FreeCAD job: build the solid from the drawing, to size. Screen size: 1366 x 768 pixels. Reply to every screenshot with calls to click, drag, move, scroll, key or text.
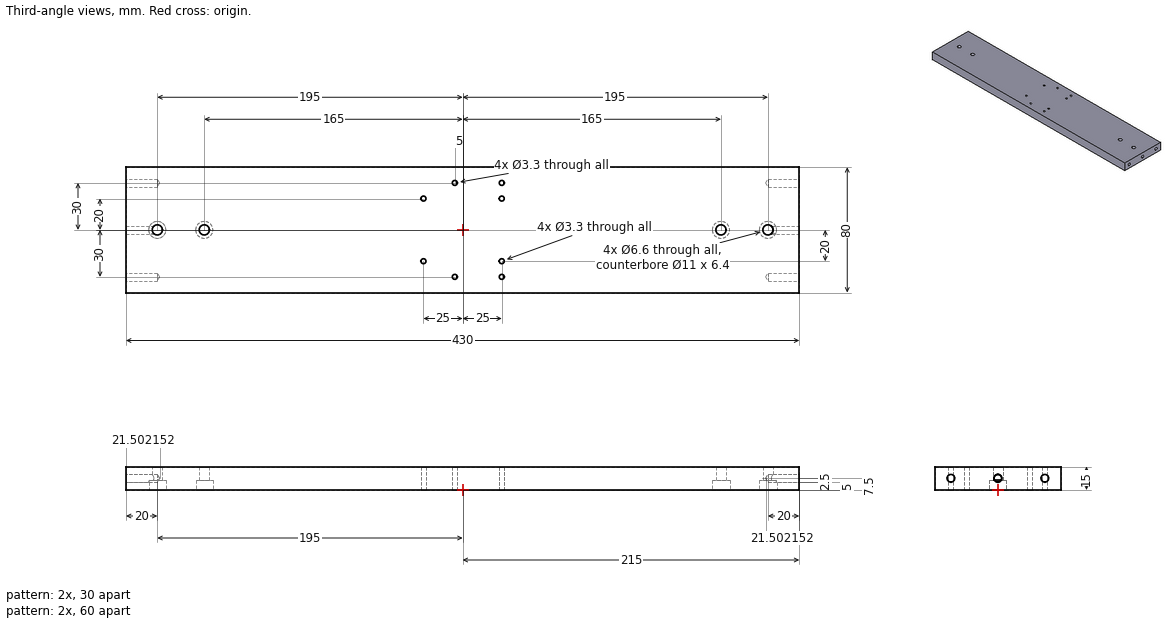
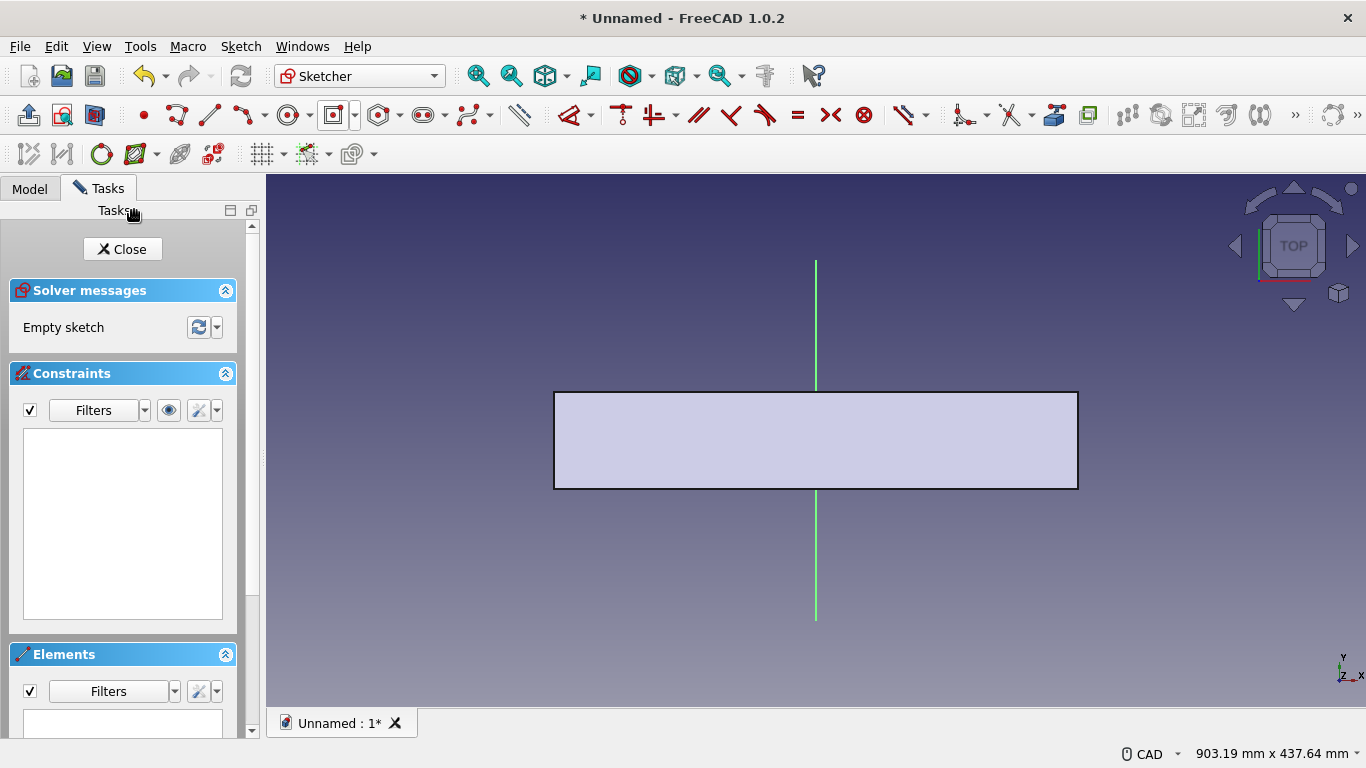
click(95, 116)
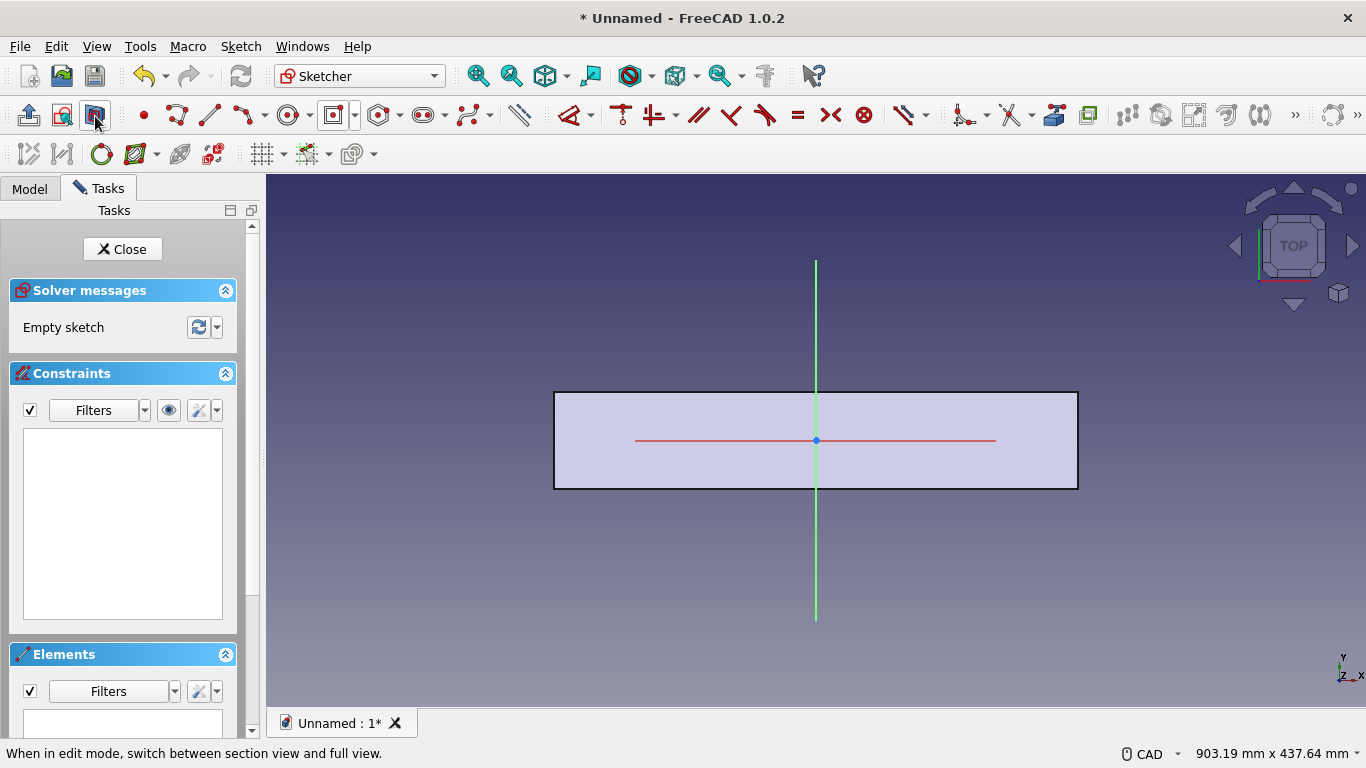
scroll(830, 440, up, 9)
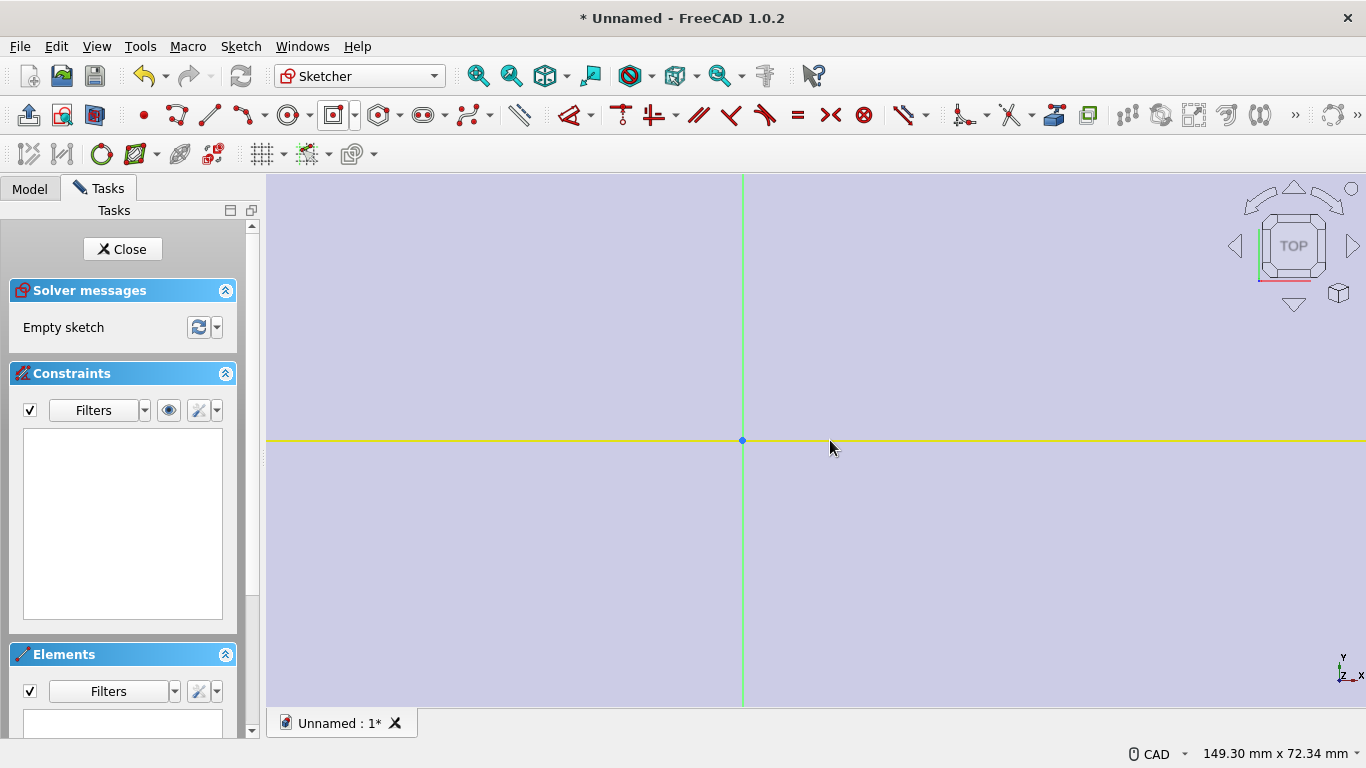
key(g)
key(c)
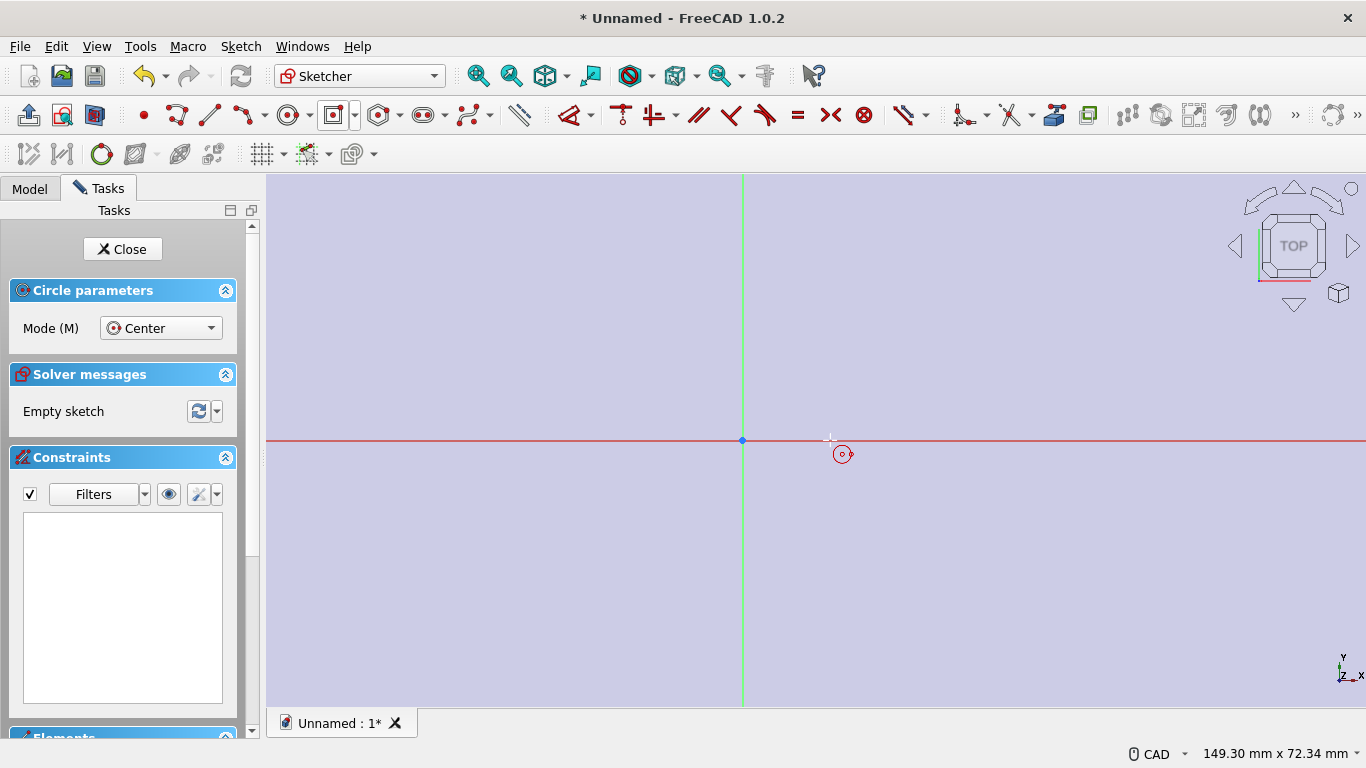
scroll(927, 588, up, 4)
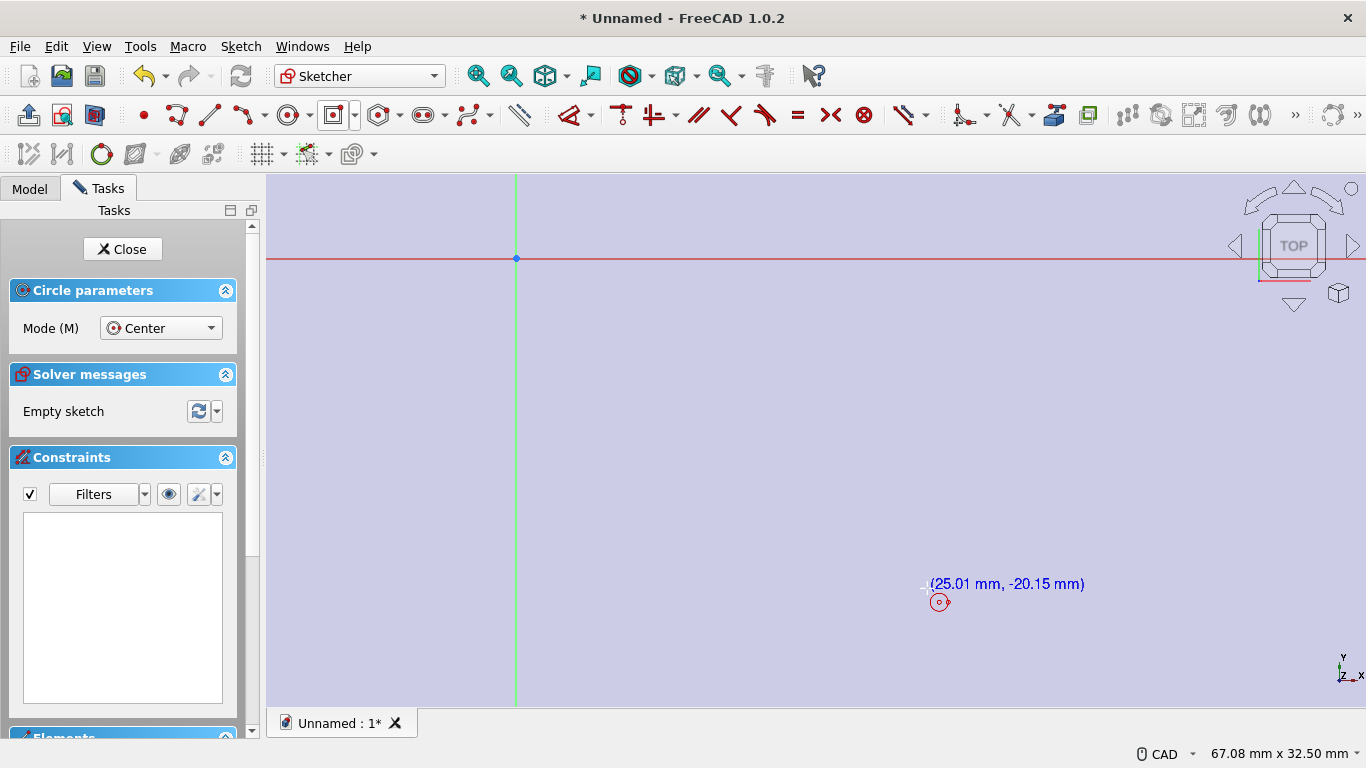
click(926, 587)
click(945, 568)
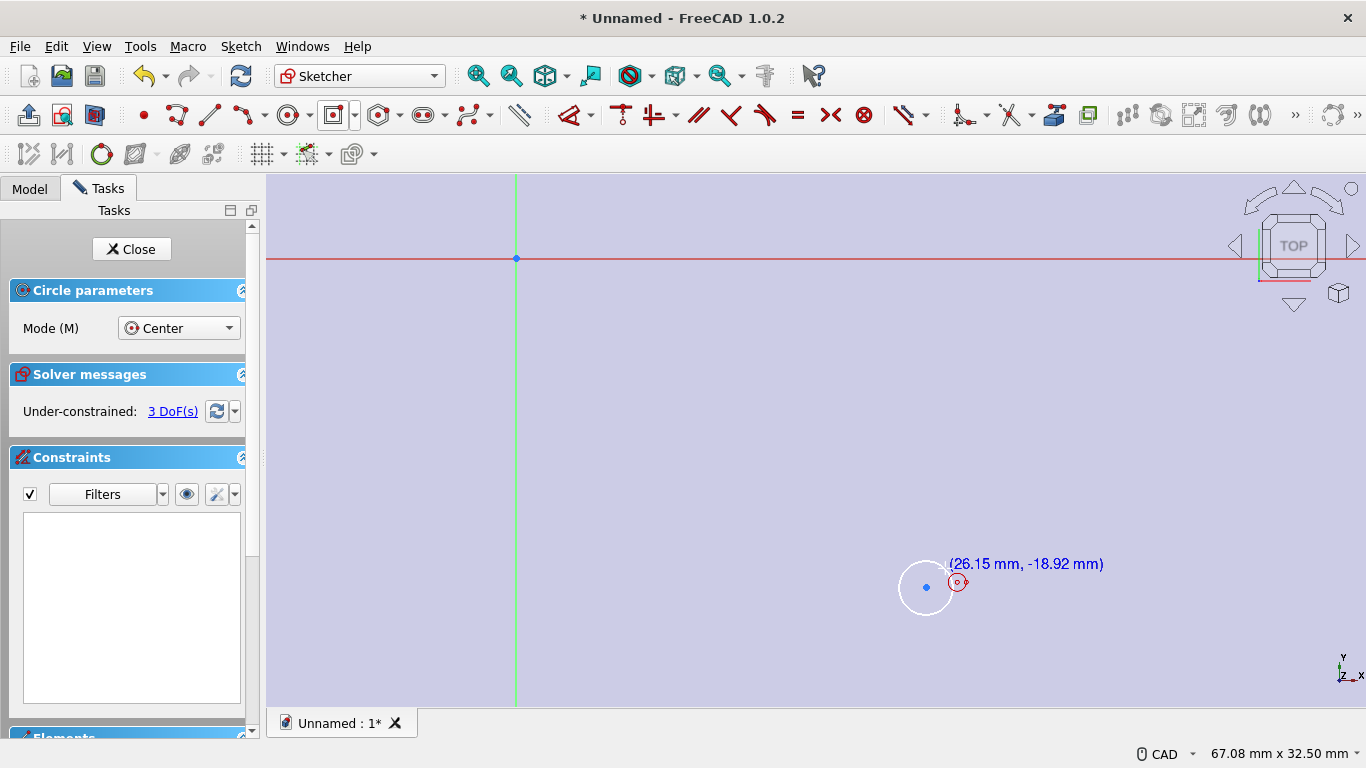
scroll(936, 589, down, 4)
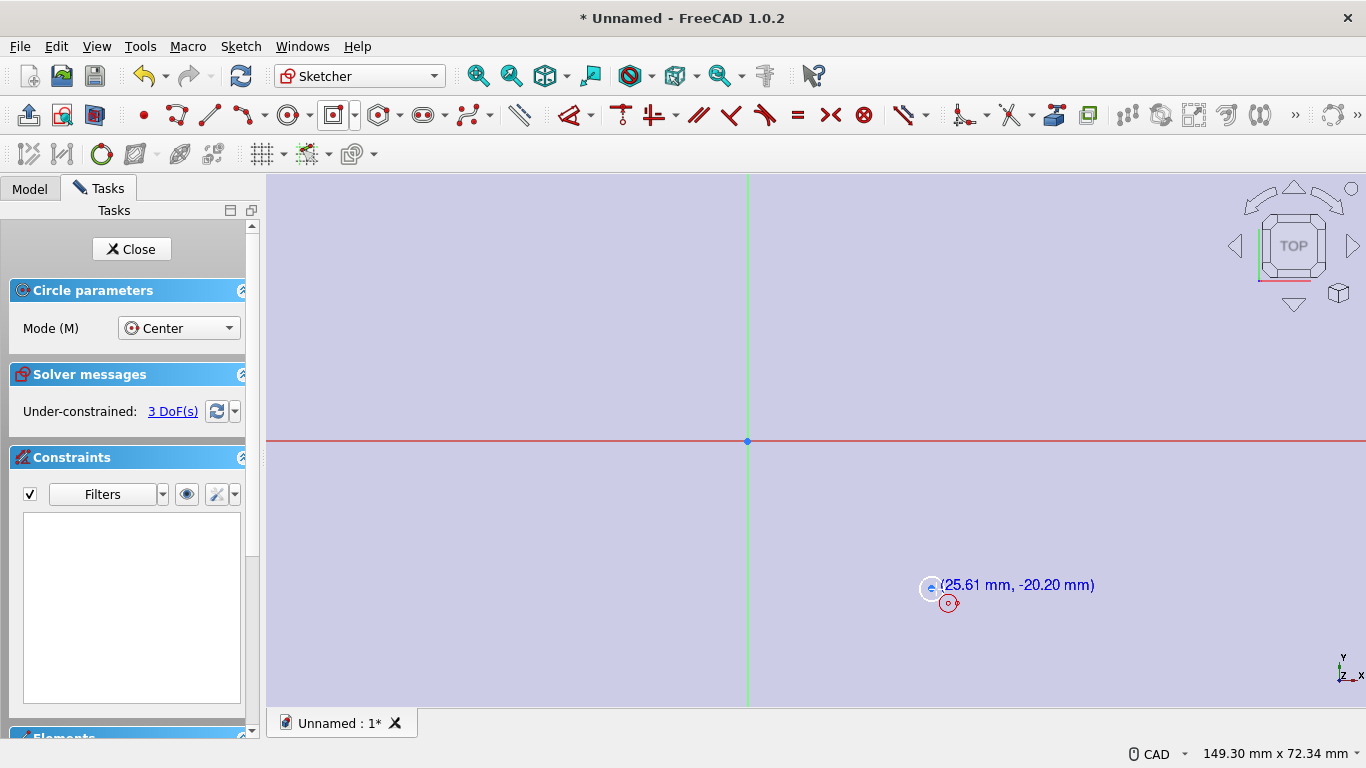
scroll(563, 588, up, 4)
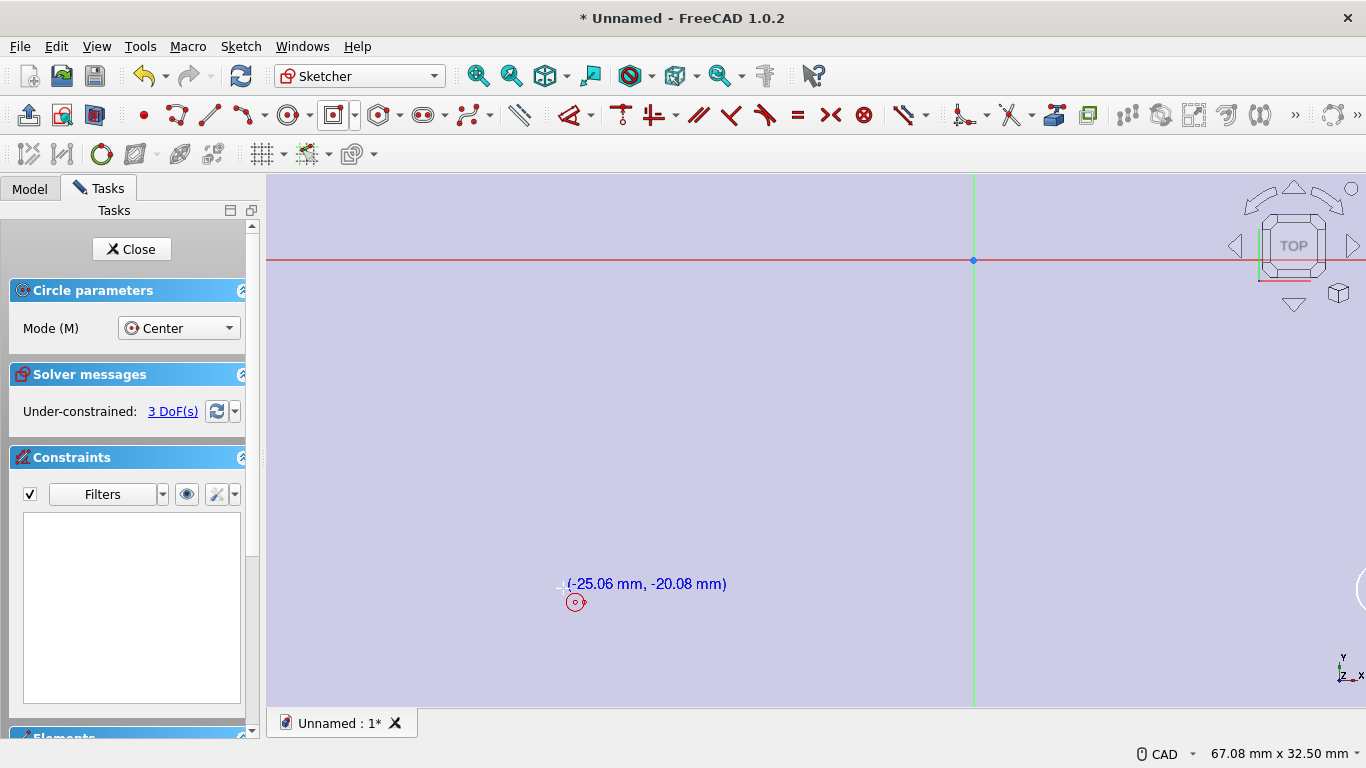
click(564, 588)
click(583, 569)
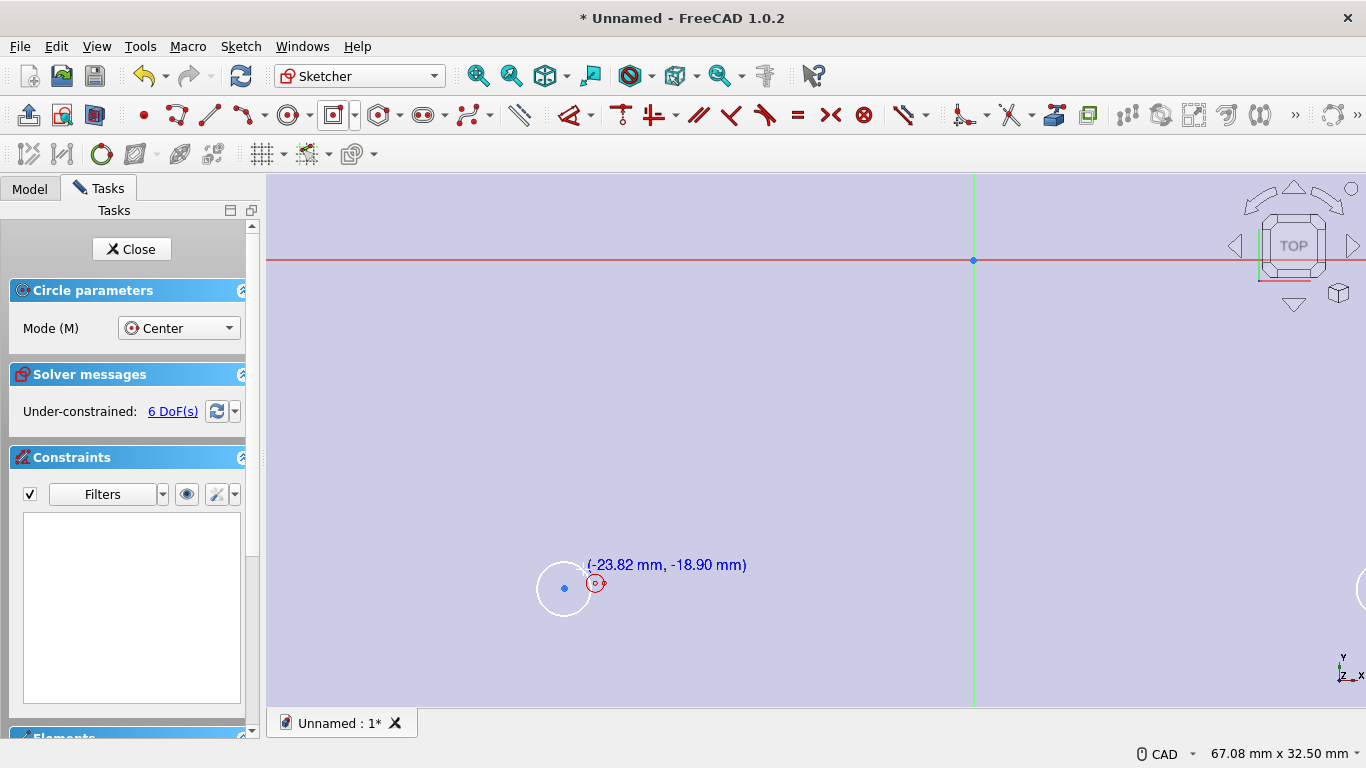
scroll(563, 588, down, 4)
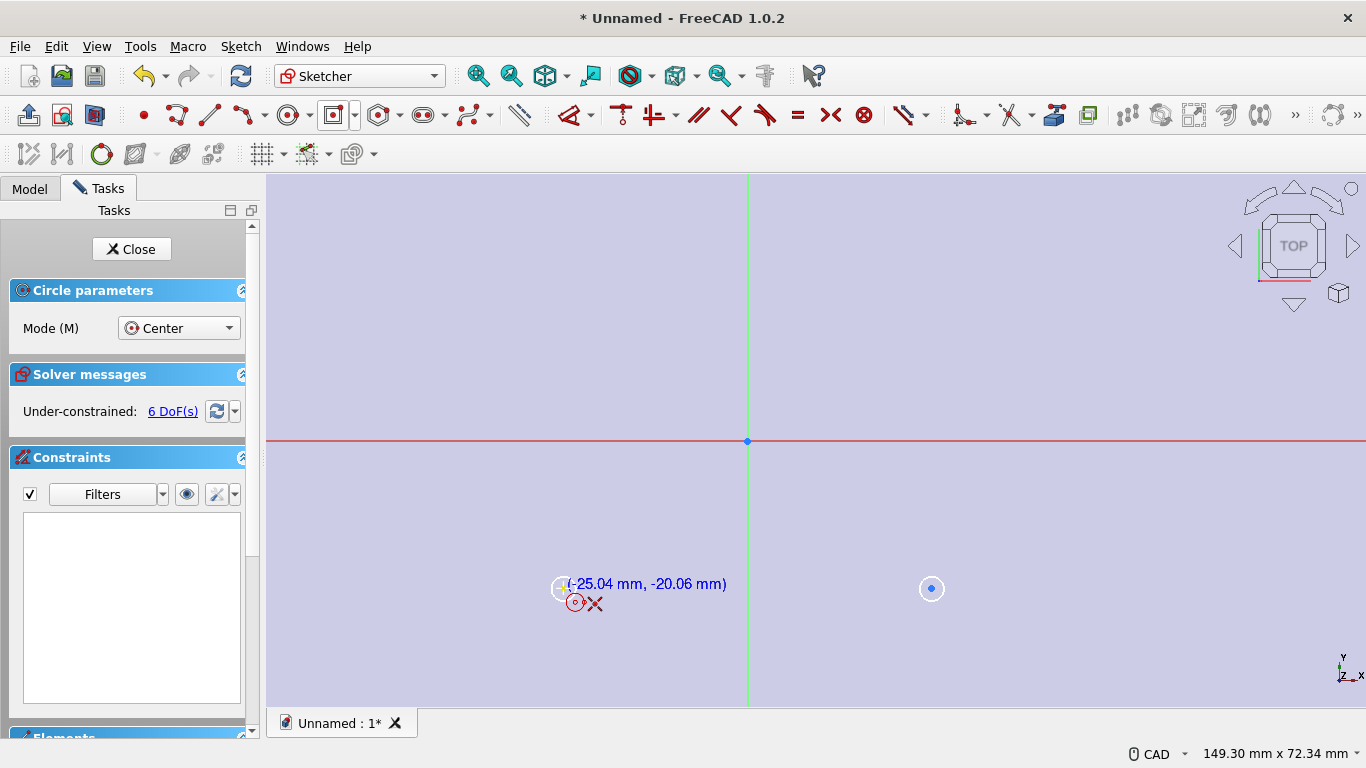
scroll(563, 294, up, 4)